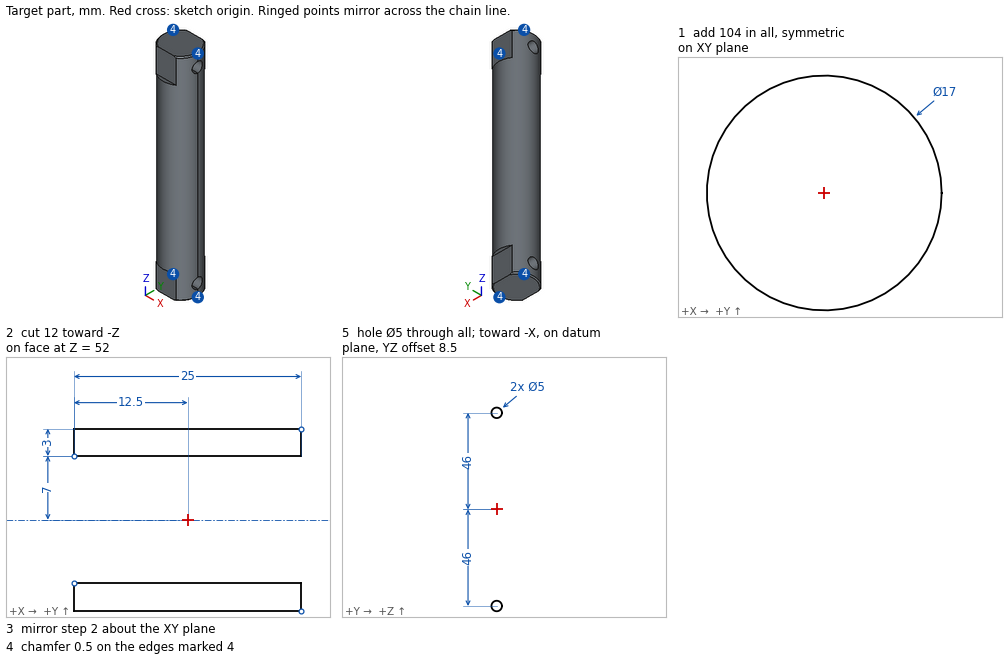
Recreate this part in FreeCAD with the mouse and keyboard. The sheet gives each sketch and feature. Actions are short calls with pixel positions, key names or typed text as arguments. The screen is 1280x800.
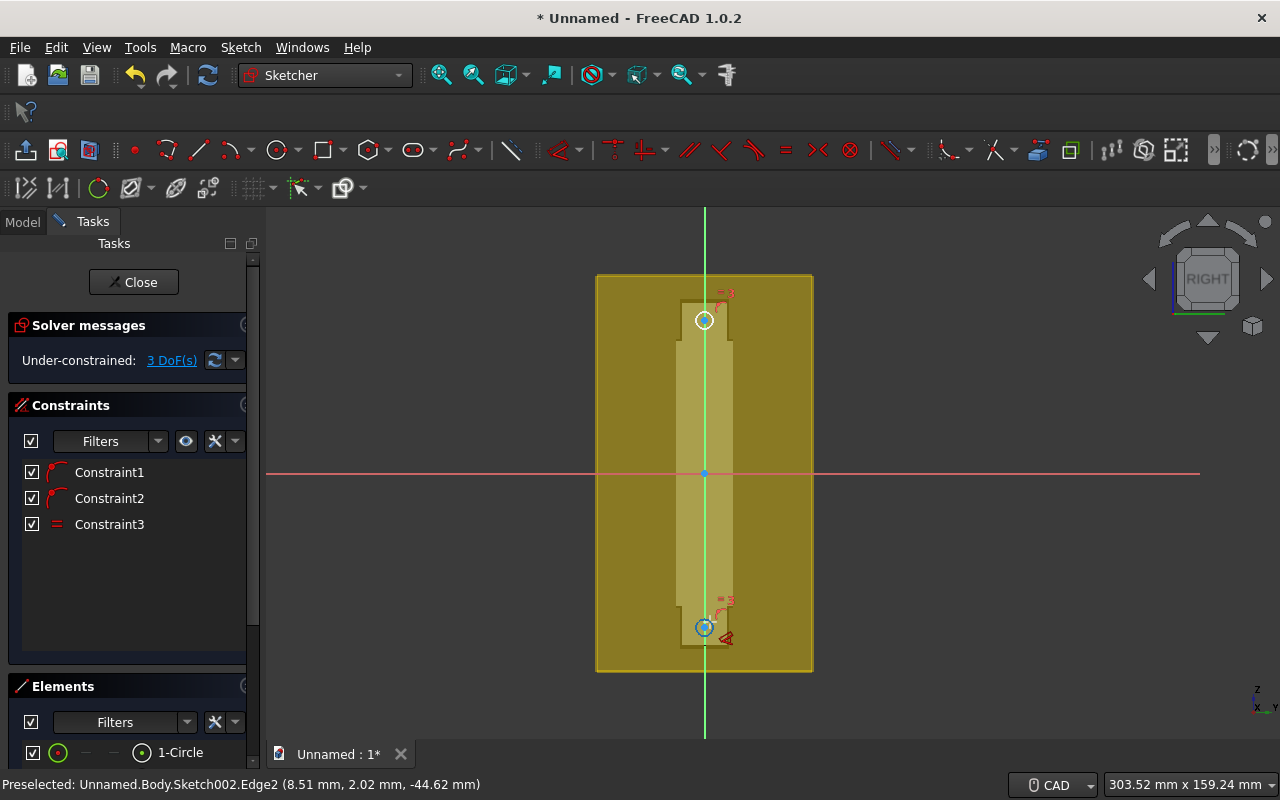
scroll(710, 315, up, 5)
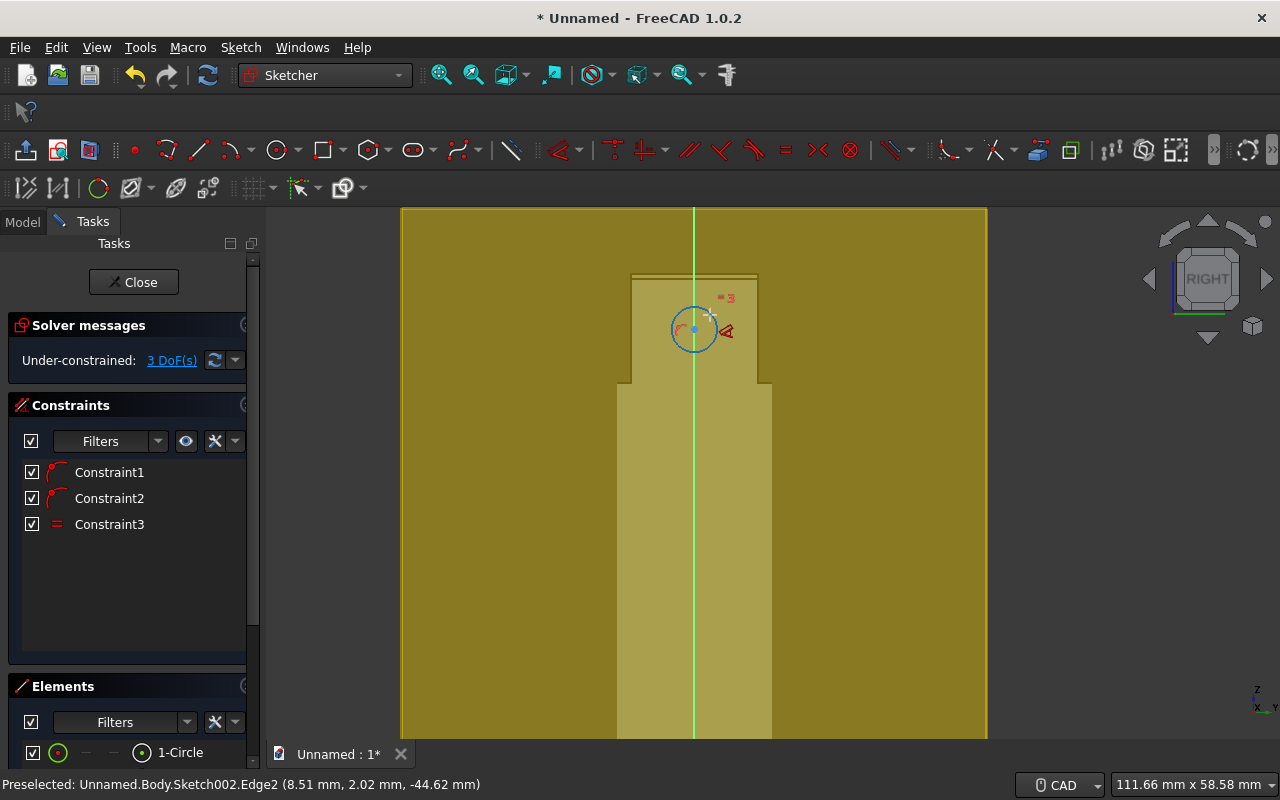
click(710, 314)
click(733, 291)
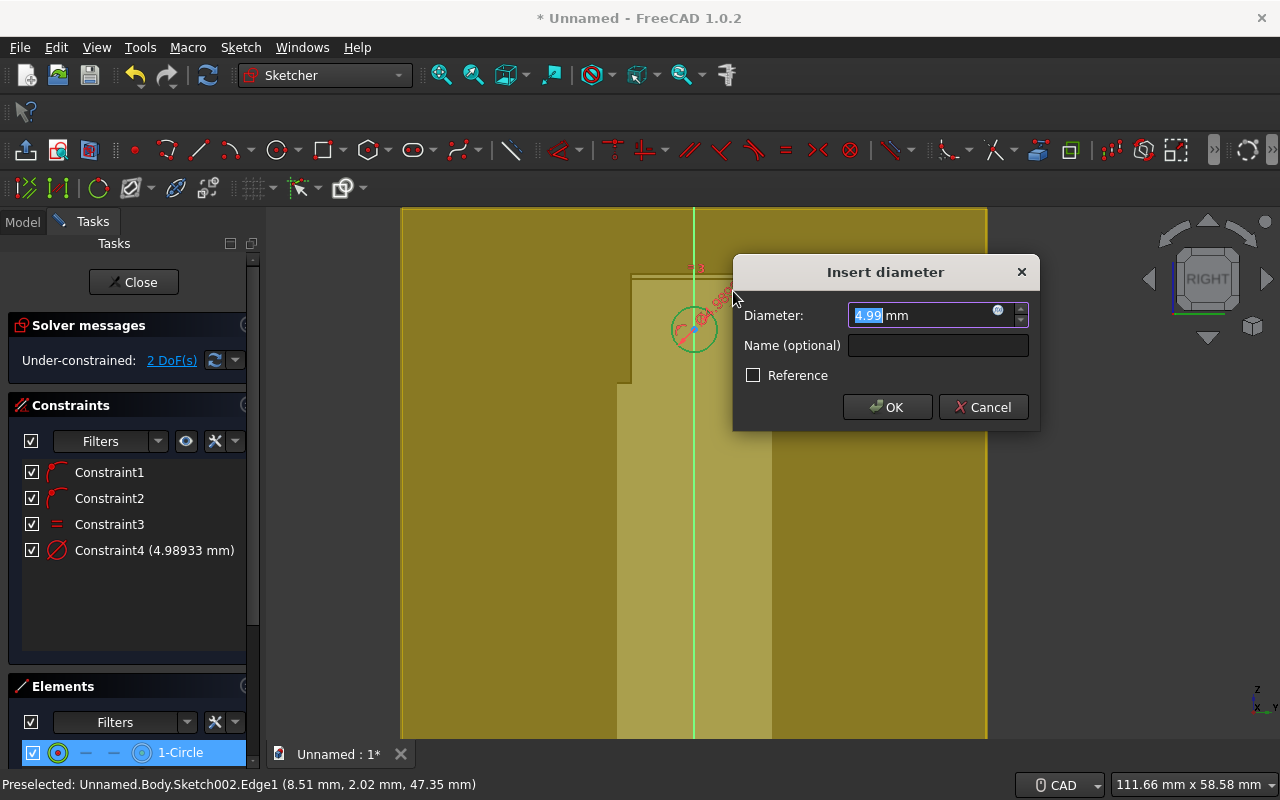
text(5)
key(Return)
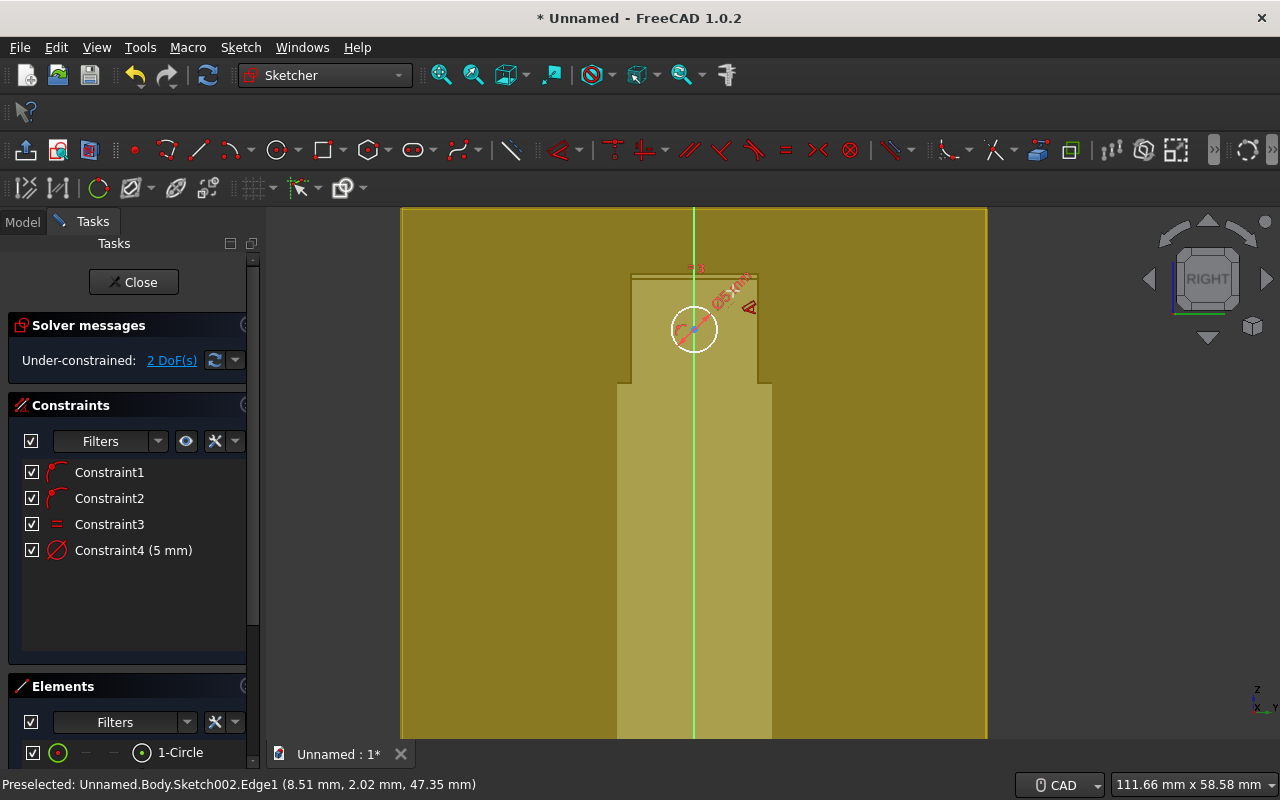
click(694, 330)
click(728, 520)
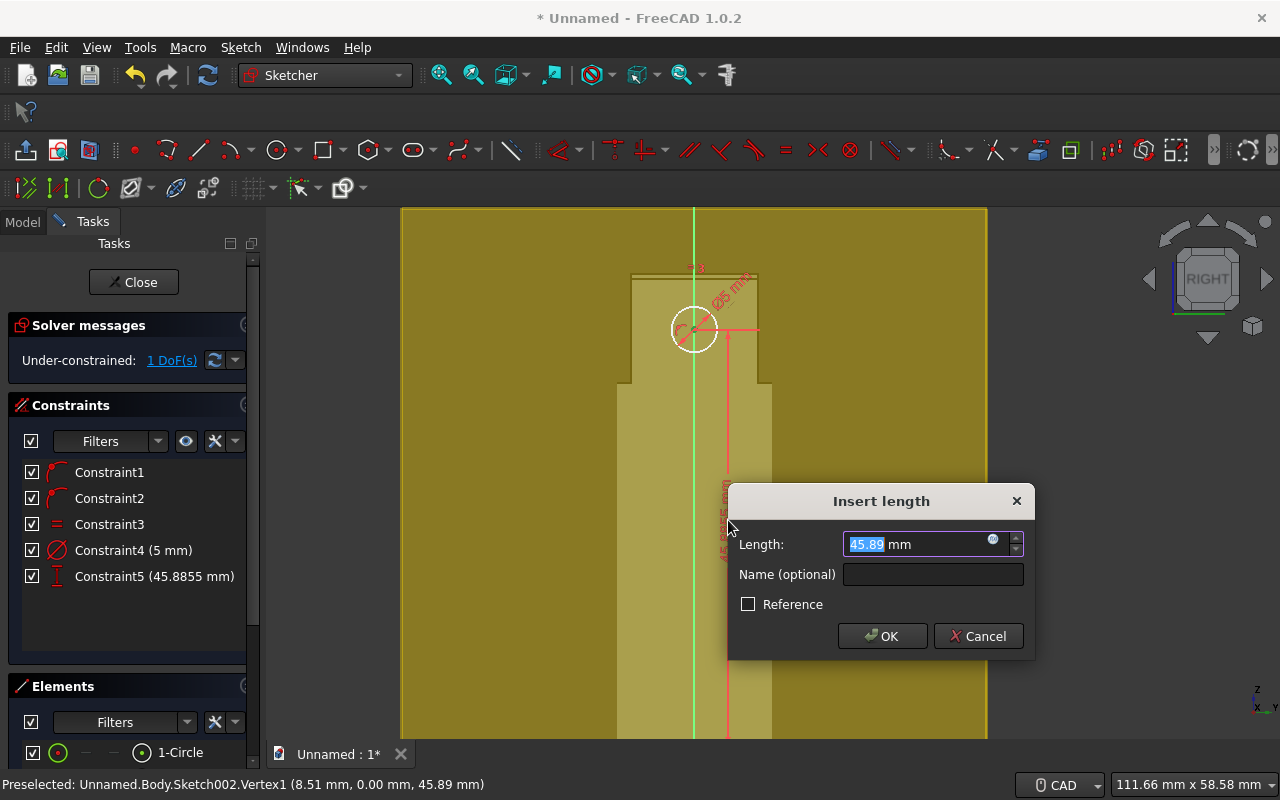
text(46)
key(Return)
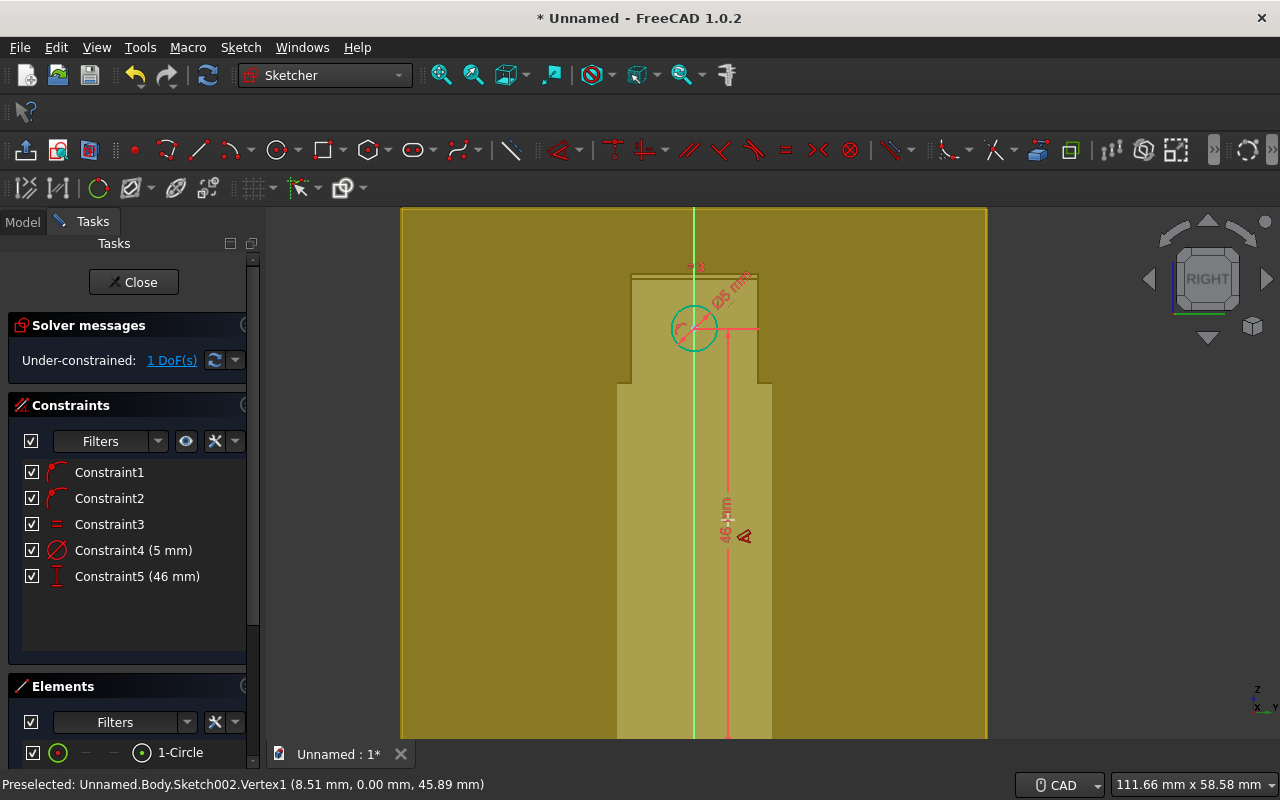
scroll(710, 314, down, 5)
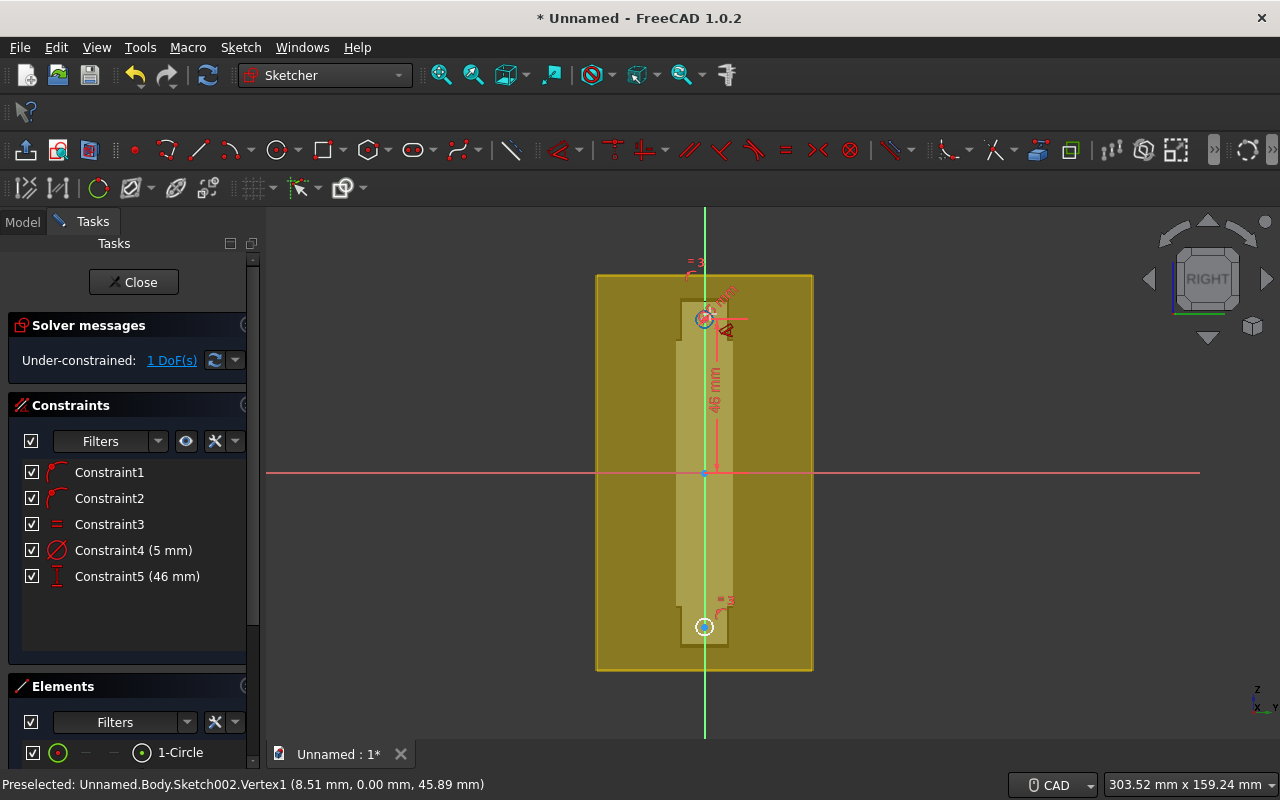
click(705, 627)
click(739, 550)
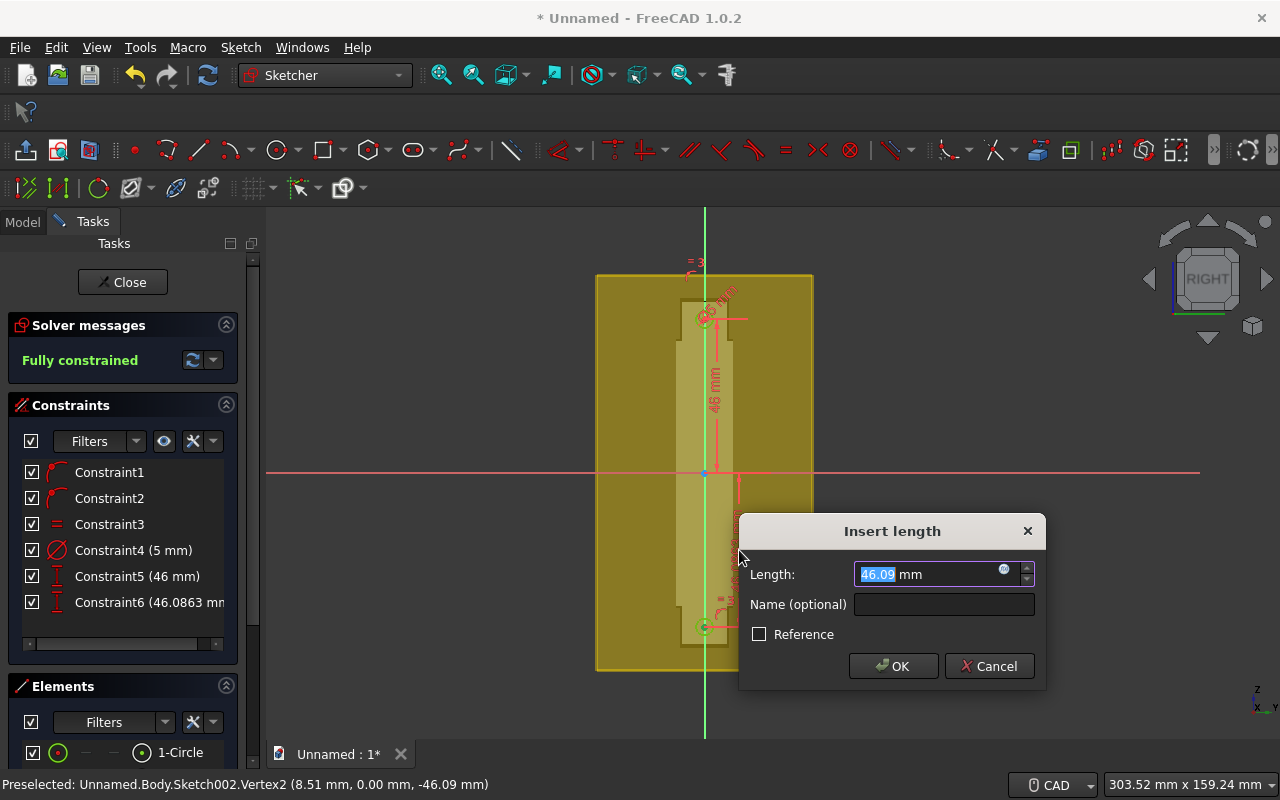
text(46)
key(Return)
key(Escape)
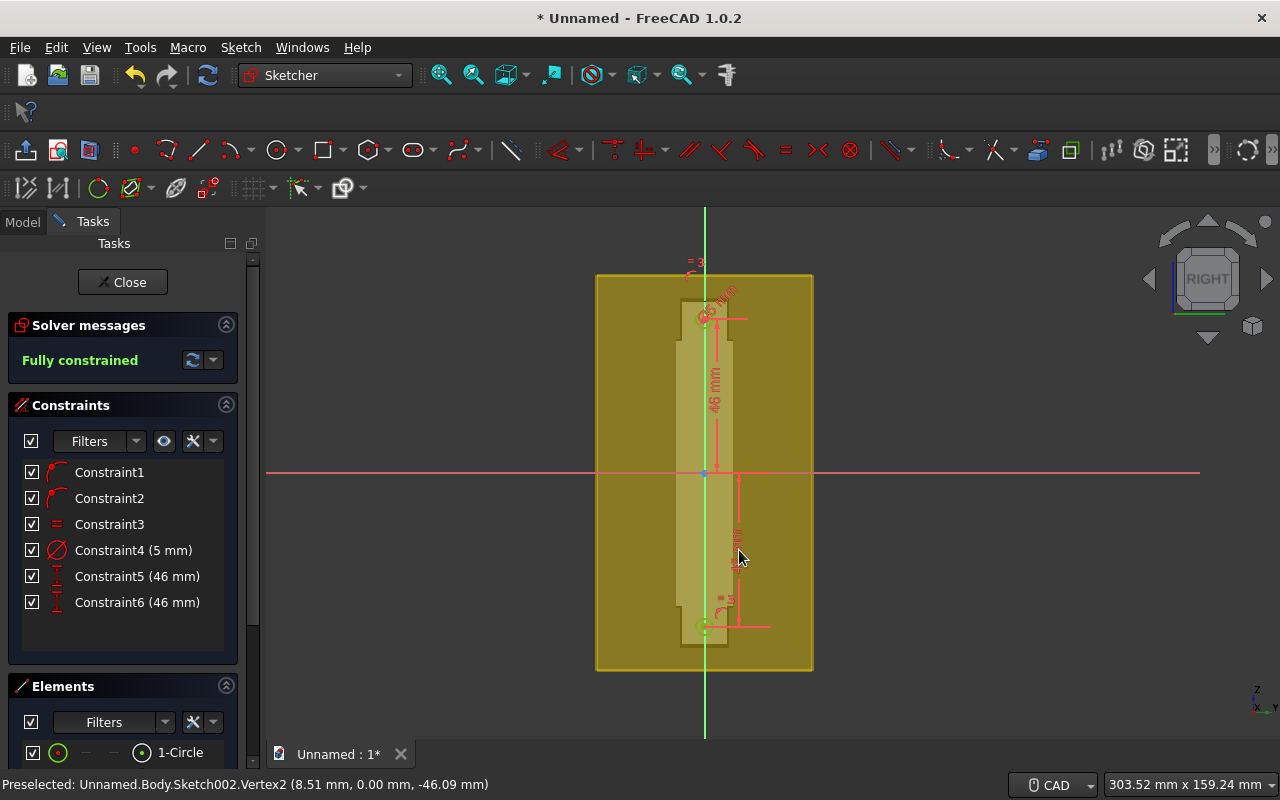
click(123, 282)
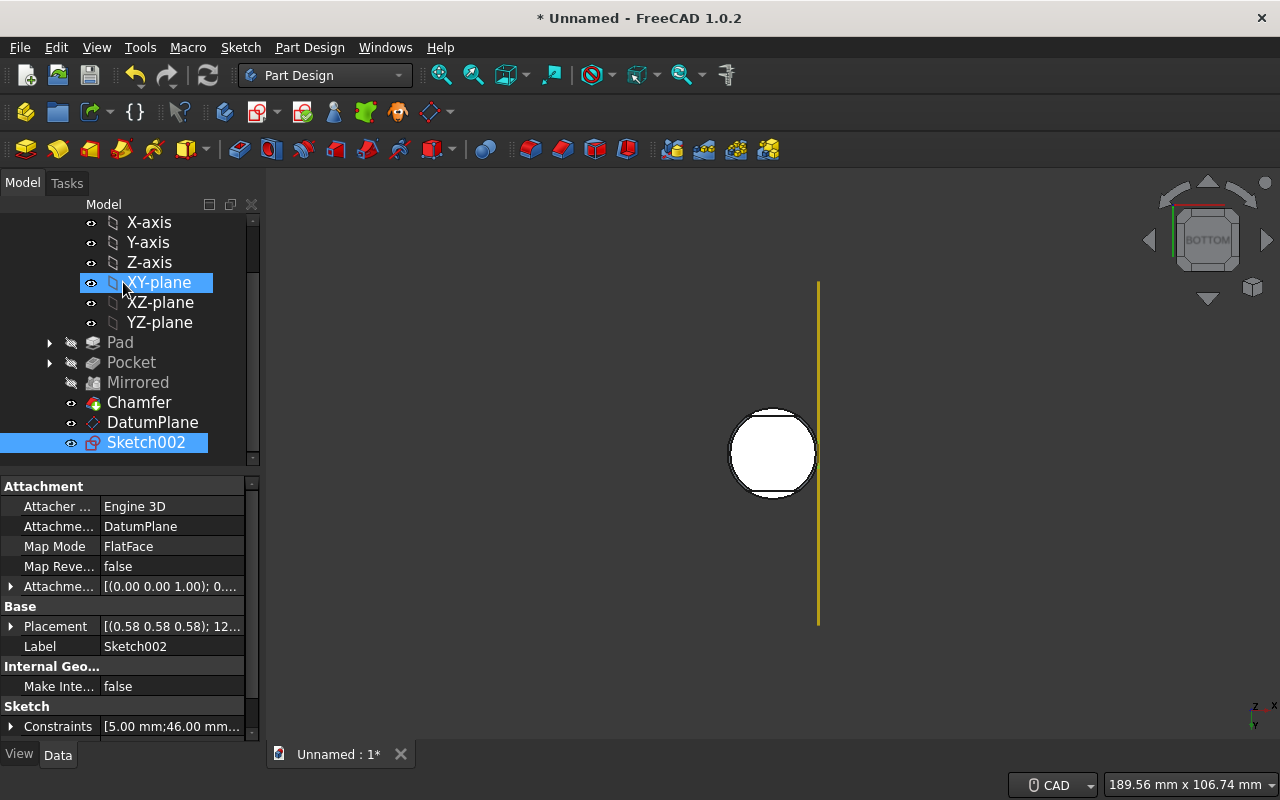
click(272, 150)